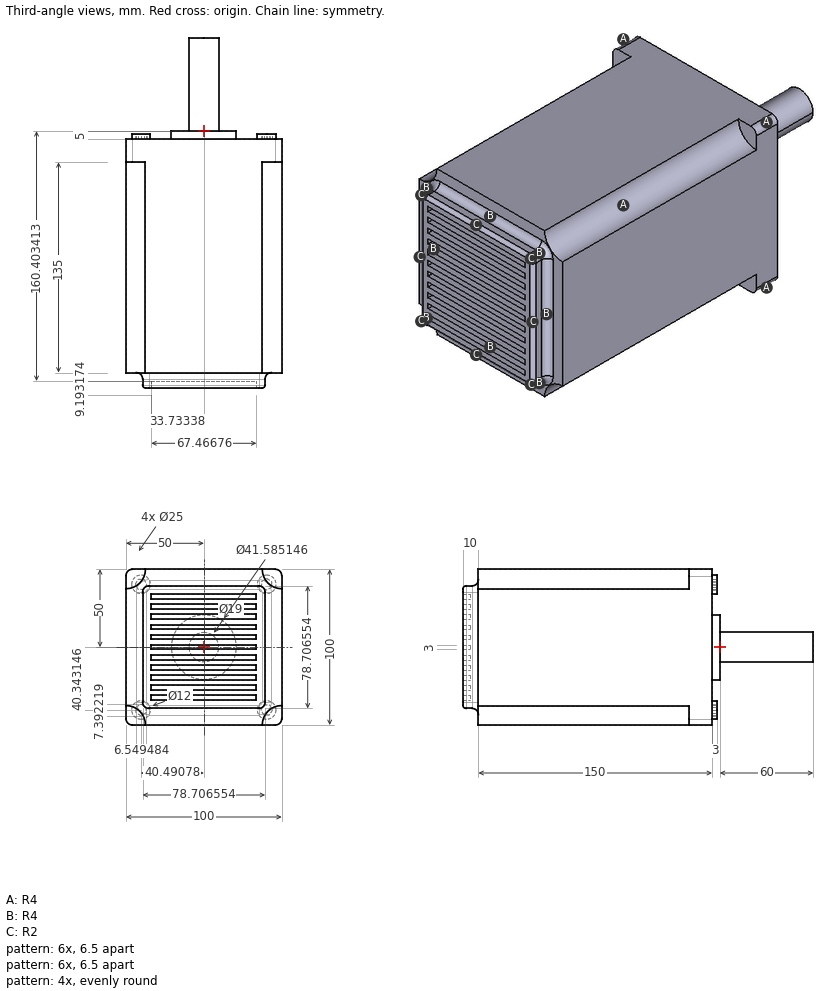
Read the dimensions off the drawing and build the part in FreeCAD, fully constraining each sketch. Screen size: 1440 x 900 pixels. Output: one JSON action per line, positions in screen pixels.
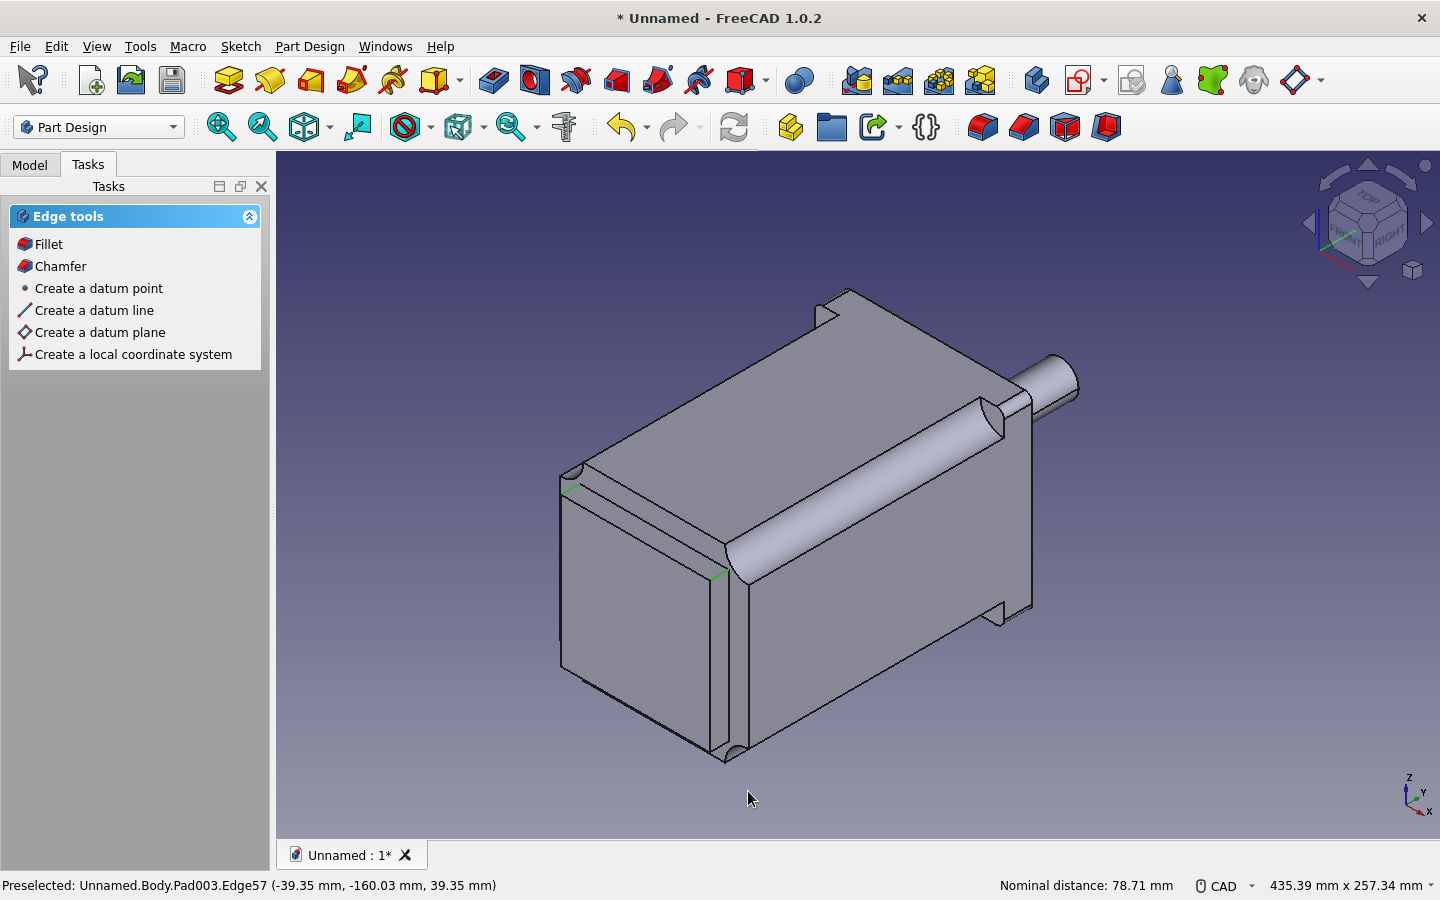
{"action": "key", "text": "1"}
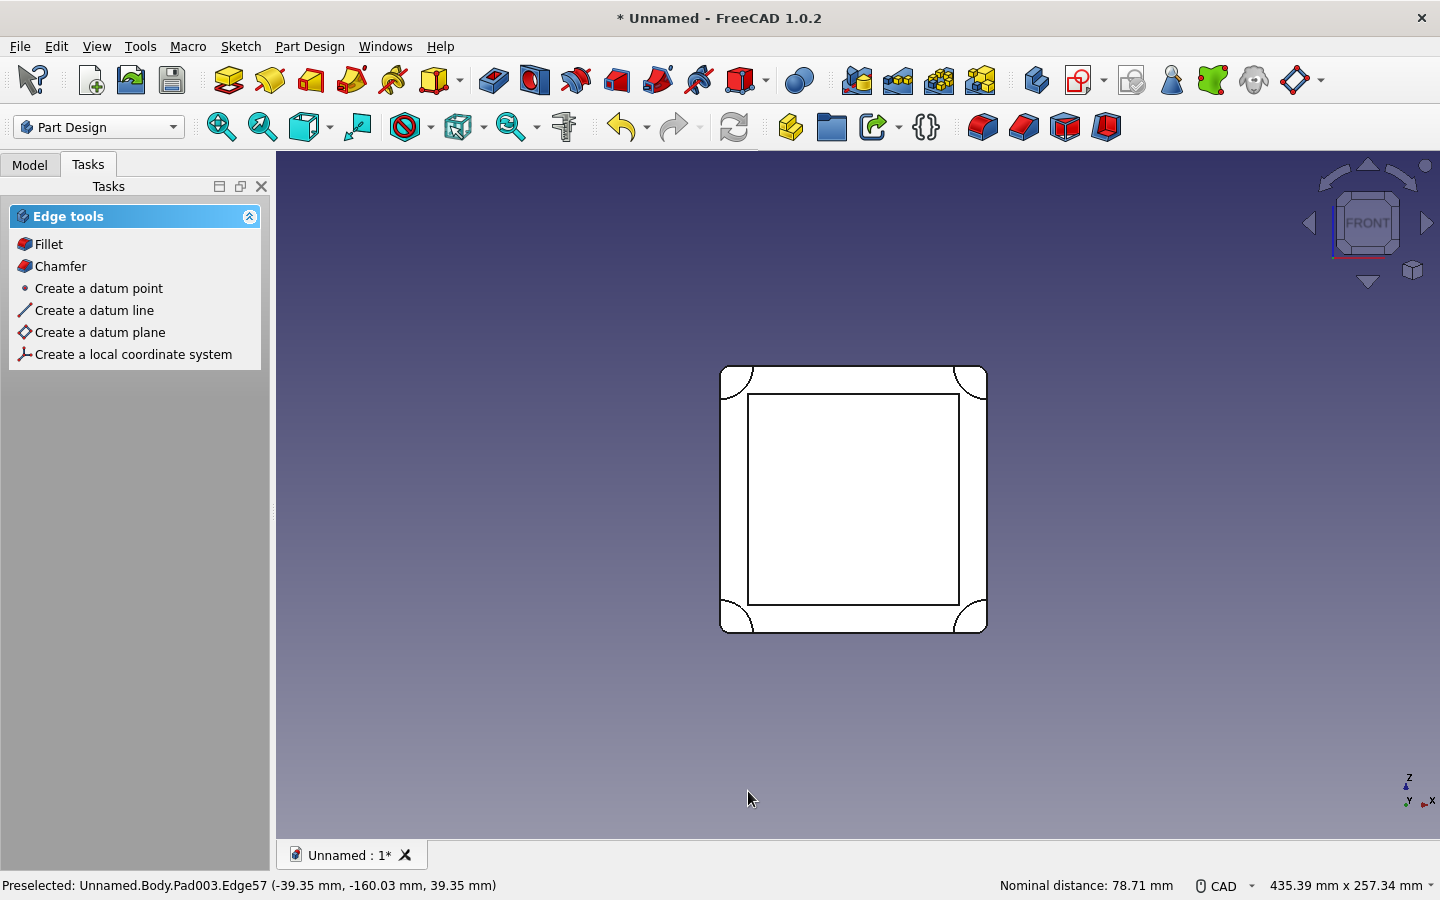
{"action": "left_click", "coordinate": [222, 128]}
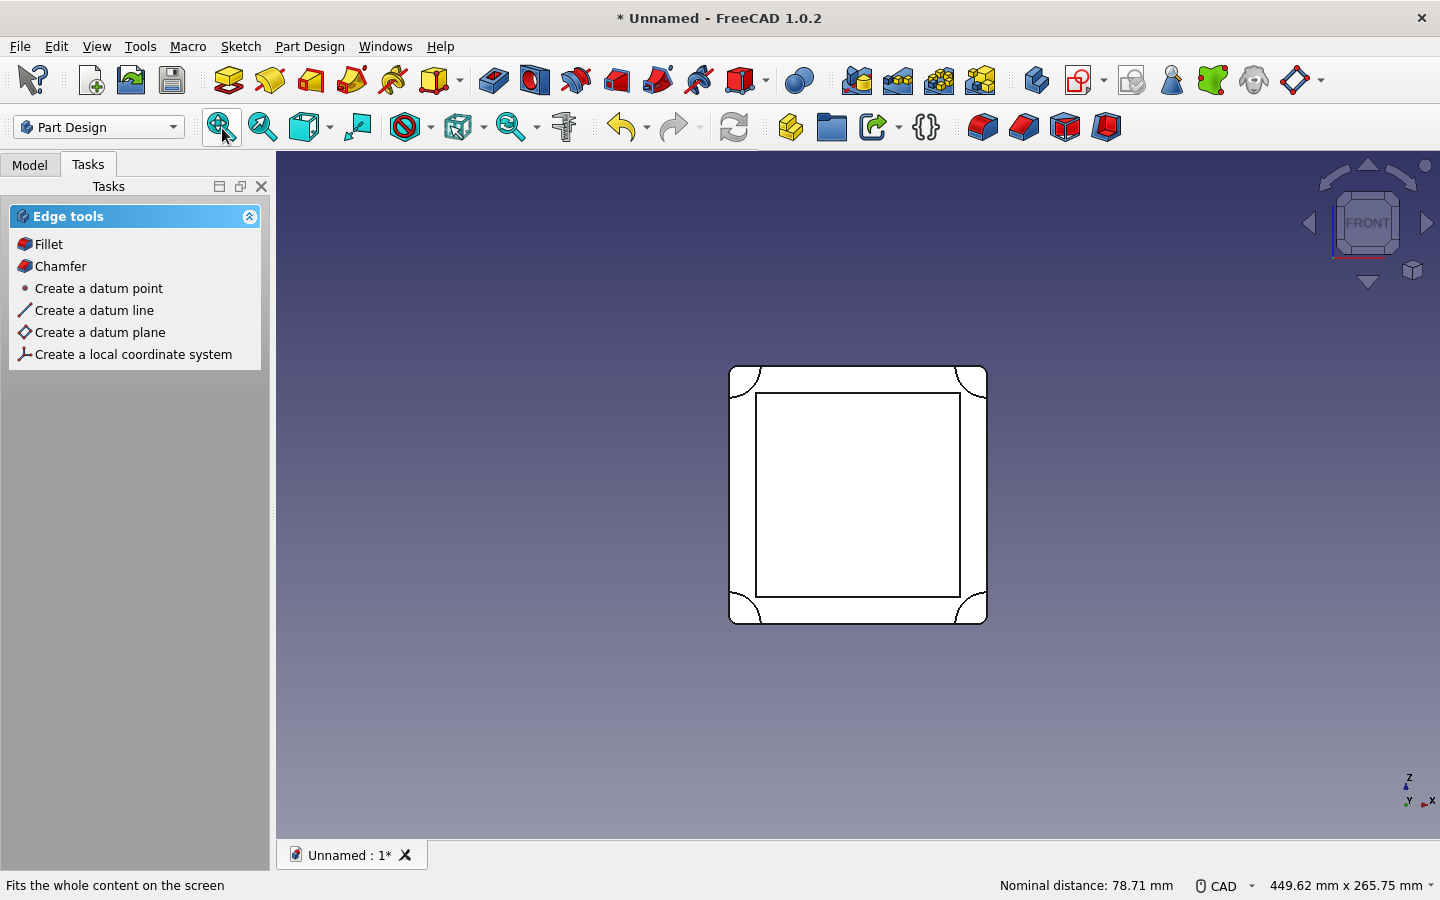
{"action": "key", "text": "3"}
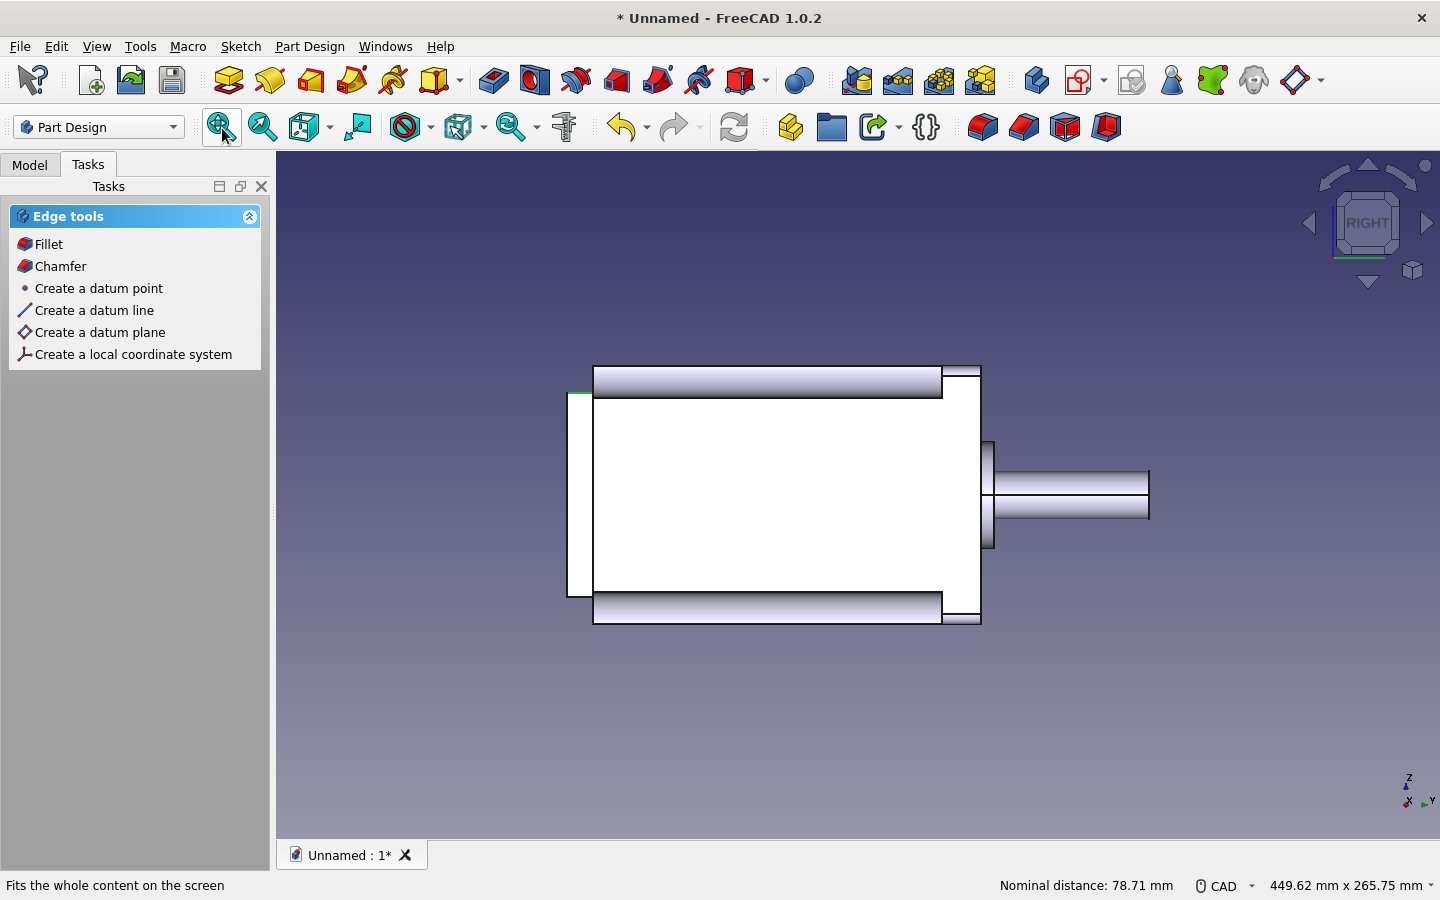
{"action": "left_click", "coordinate": [580, 596], "text": "ctrl"}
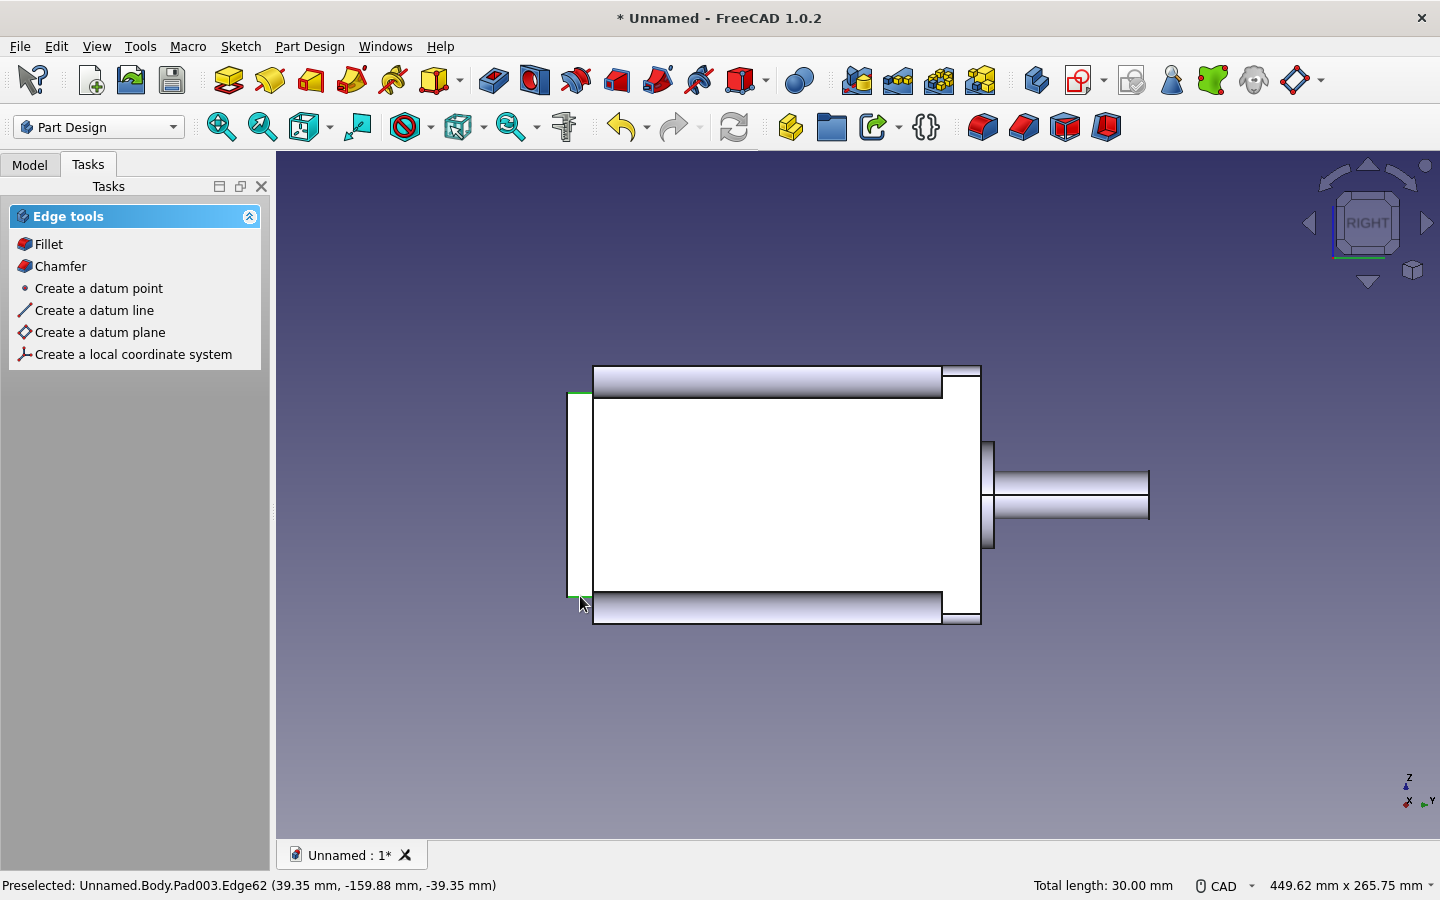
{"action": "key", "text": "5"}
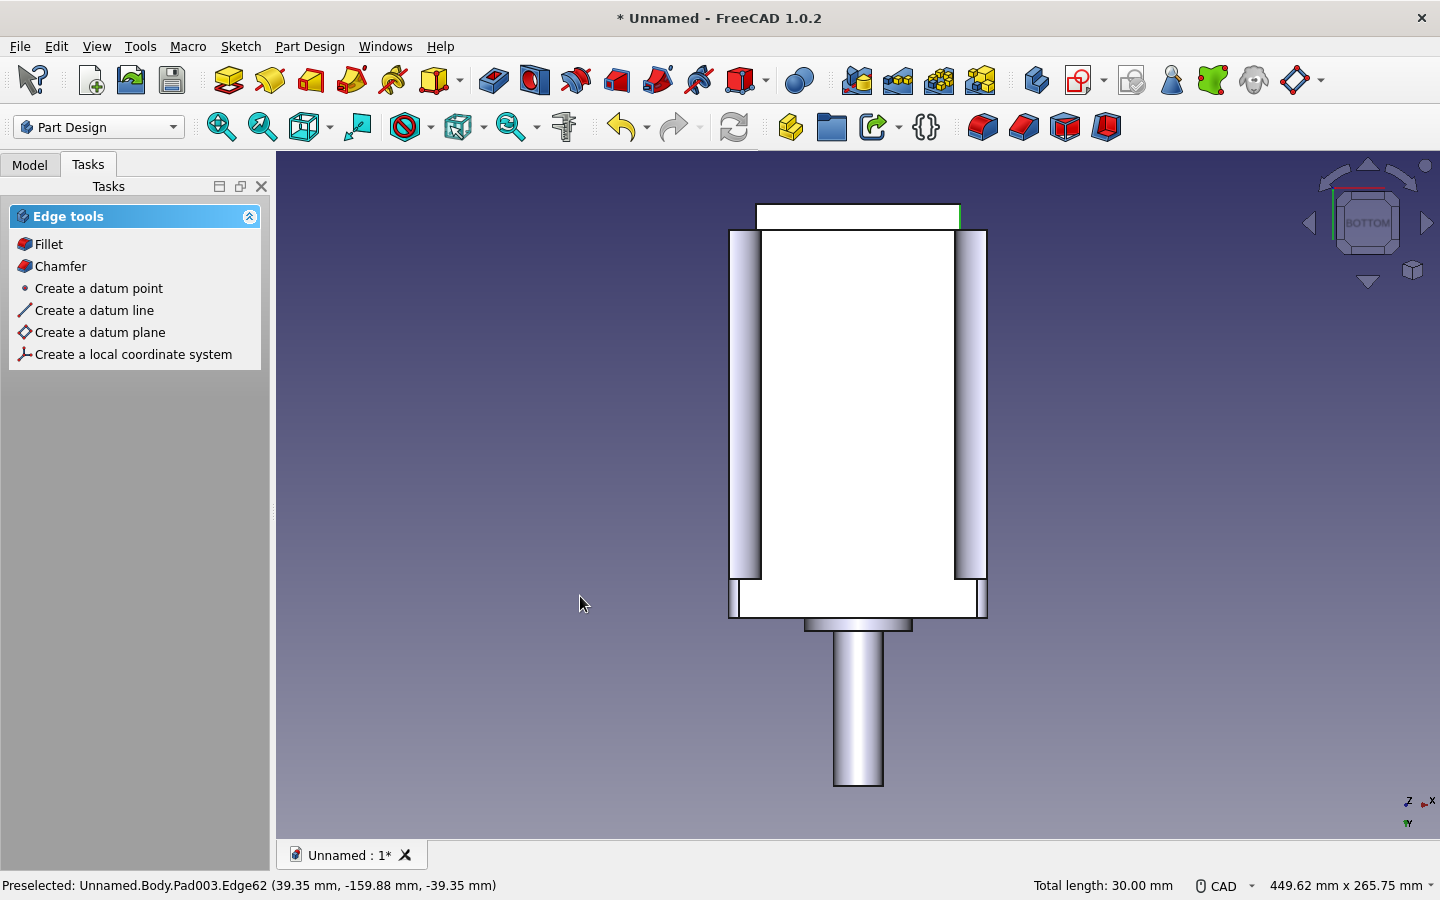
{"action": "left_click", "coordinate": [756, 216], "text": "ctrl"}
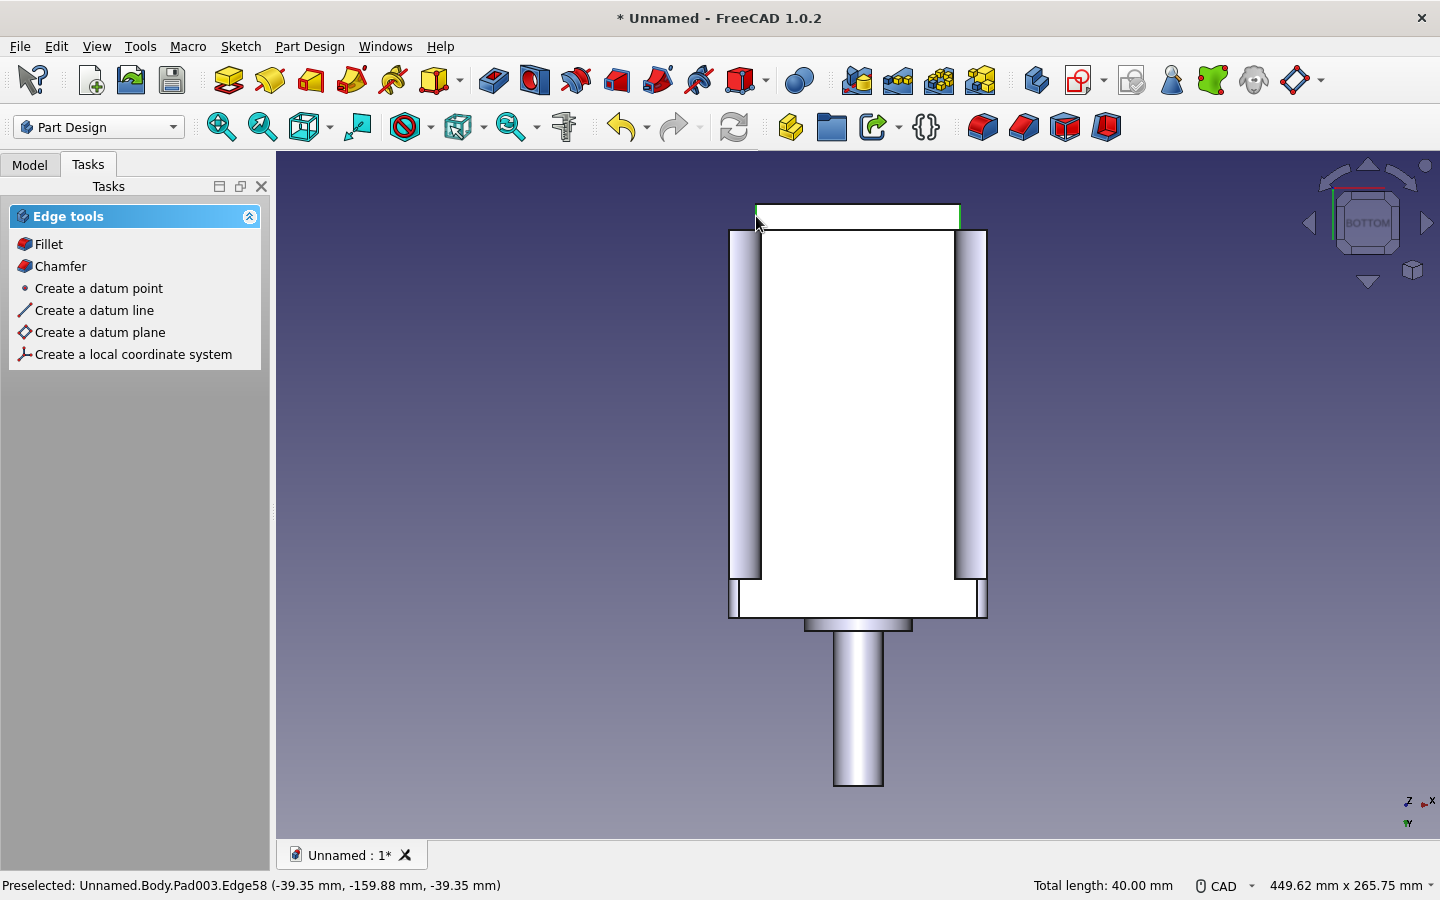
{"action": "key", "text": "4"}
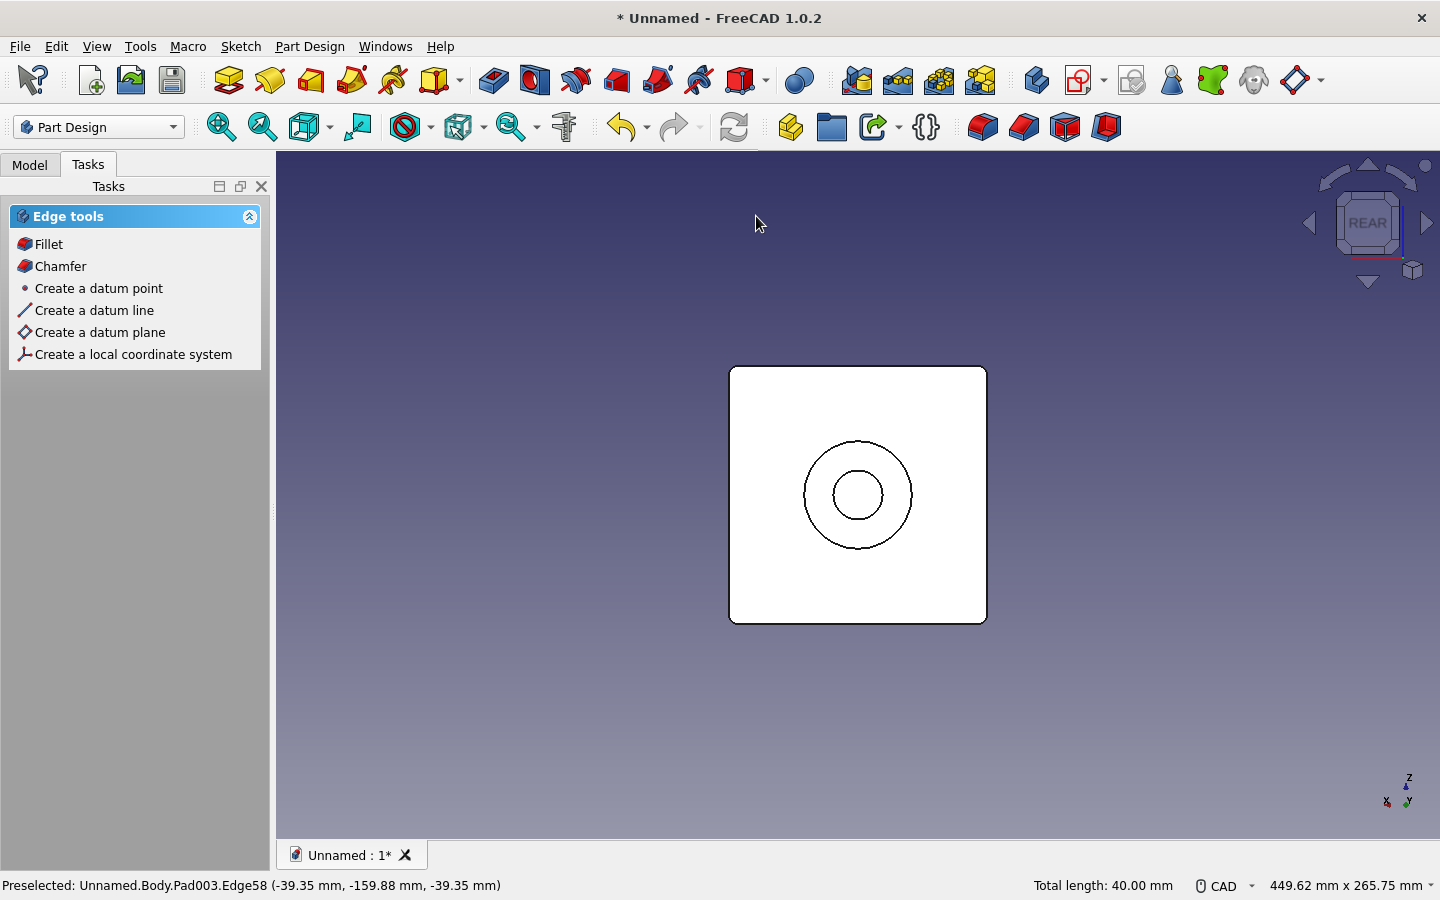
{"action": "left_click", "coordinate": [222, 128]}